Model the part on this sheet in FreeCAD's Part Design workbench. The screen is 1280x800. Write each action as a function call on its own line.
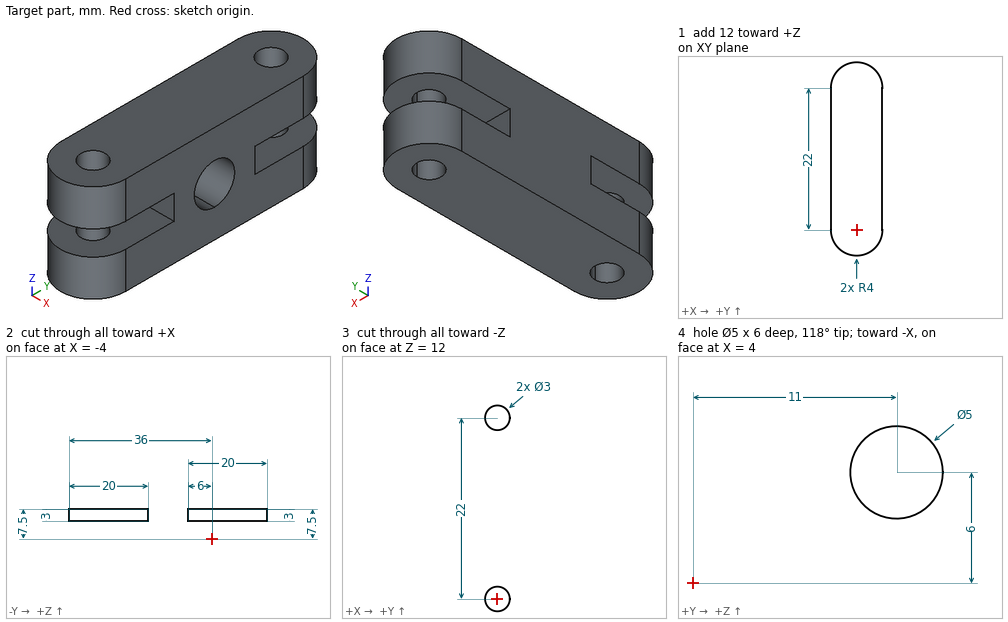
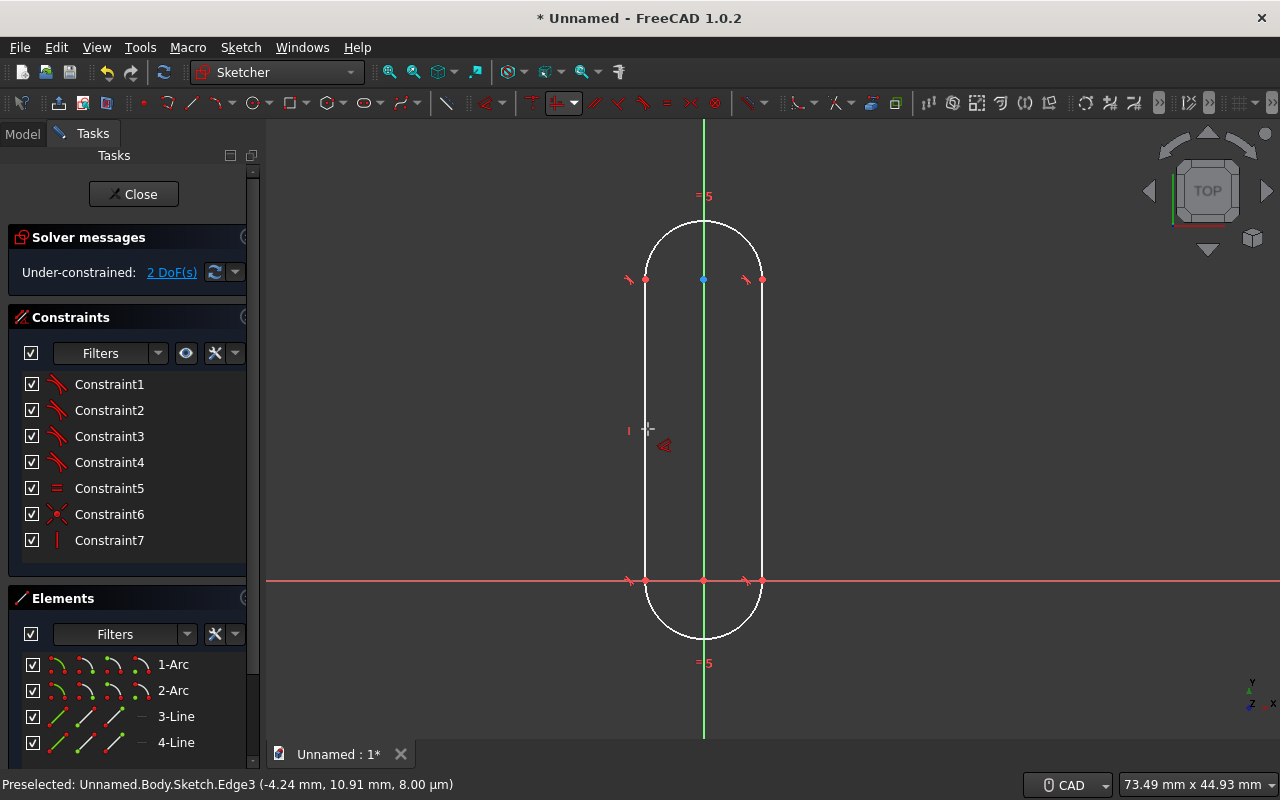
click(669, 628)
click(650, 654)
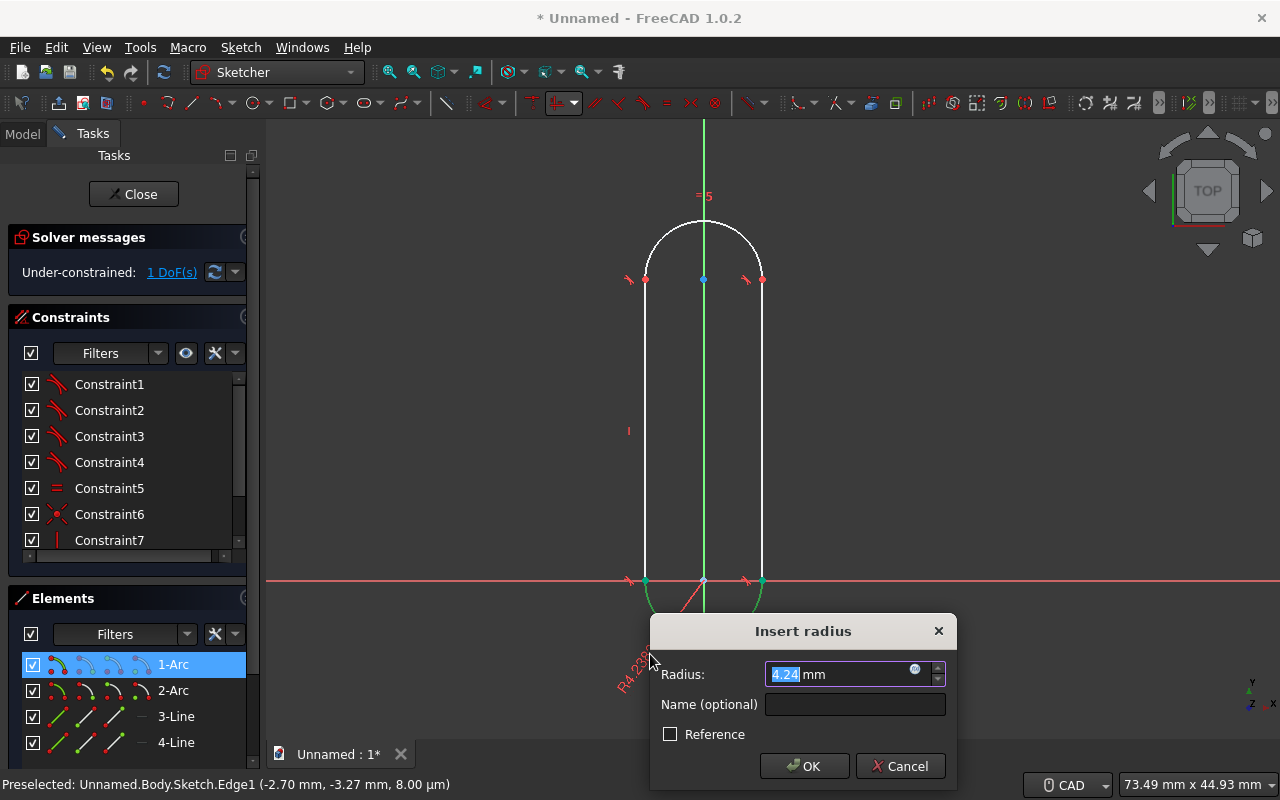
text(4)
key(Return)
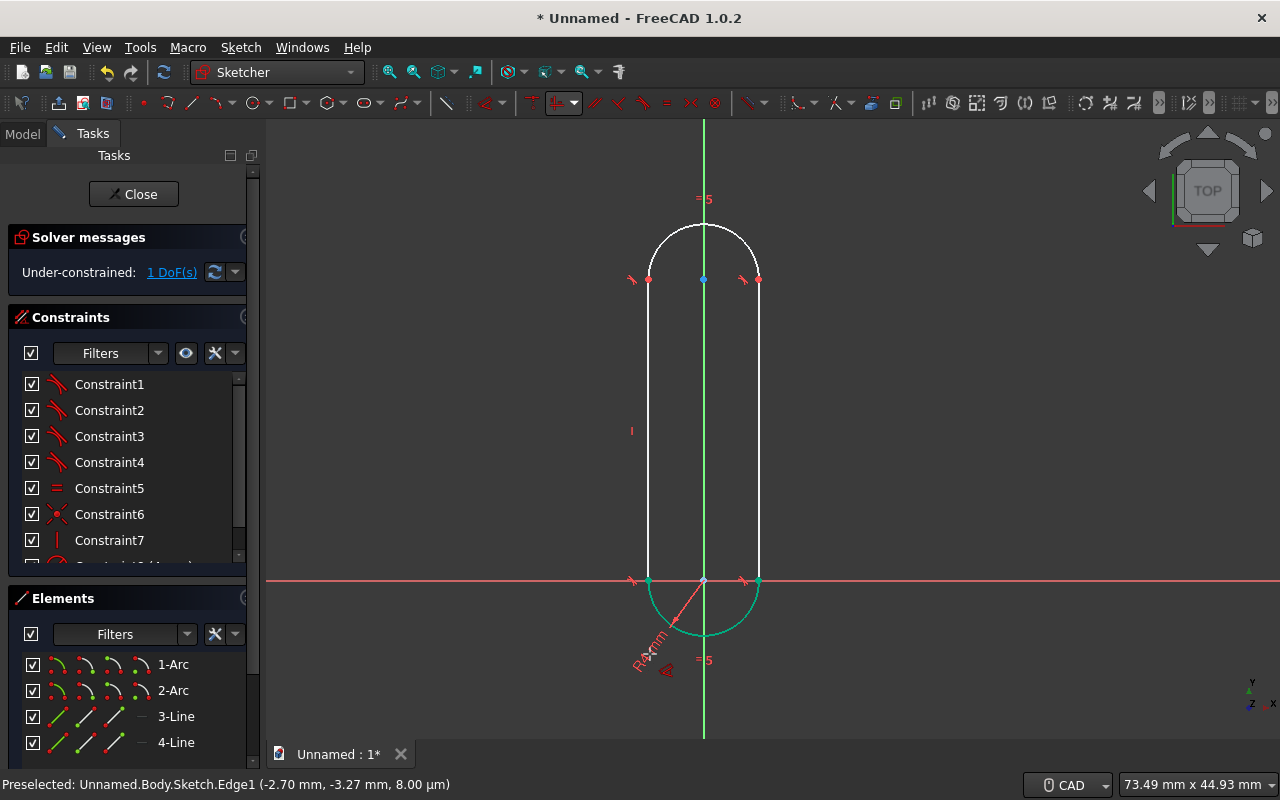
click(648, 490)
click(614, 430)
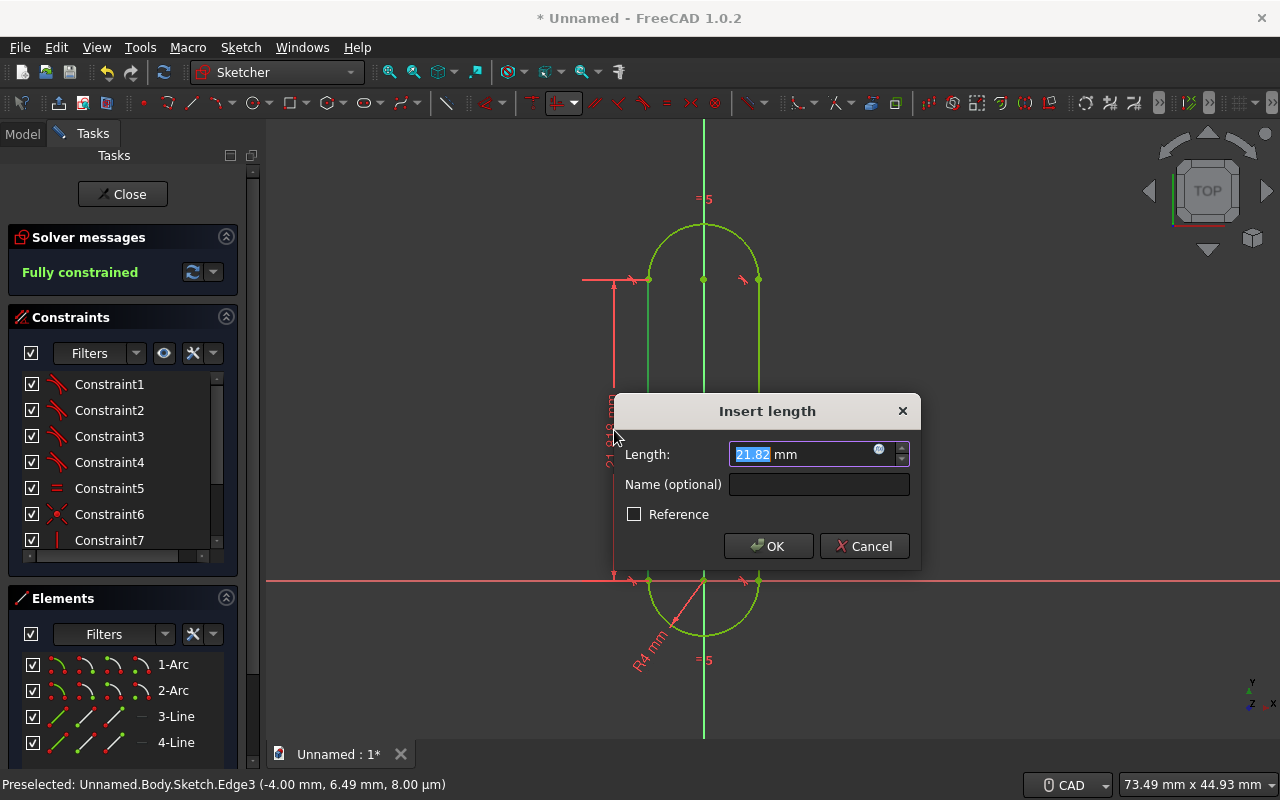
text(22)
key(Return)
key(Escape)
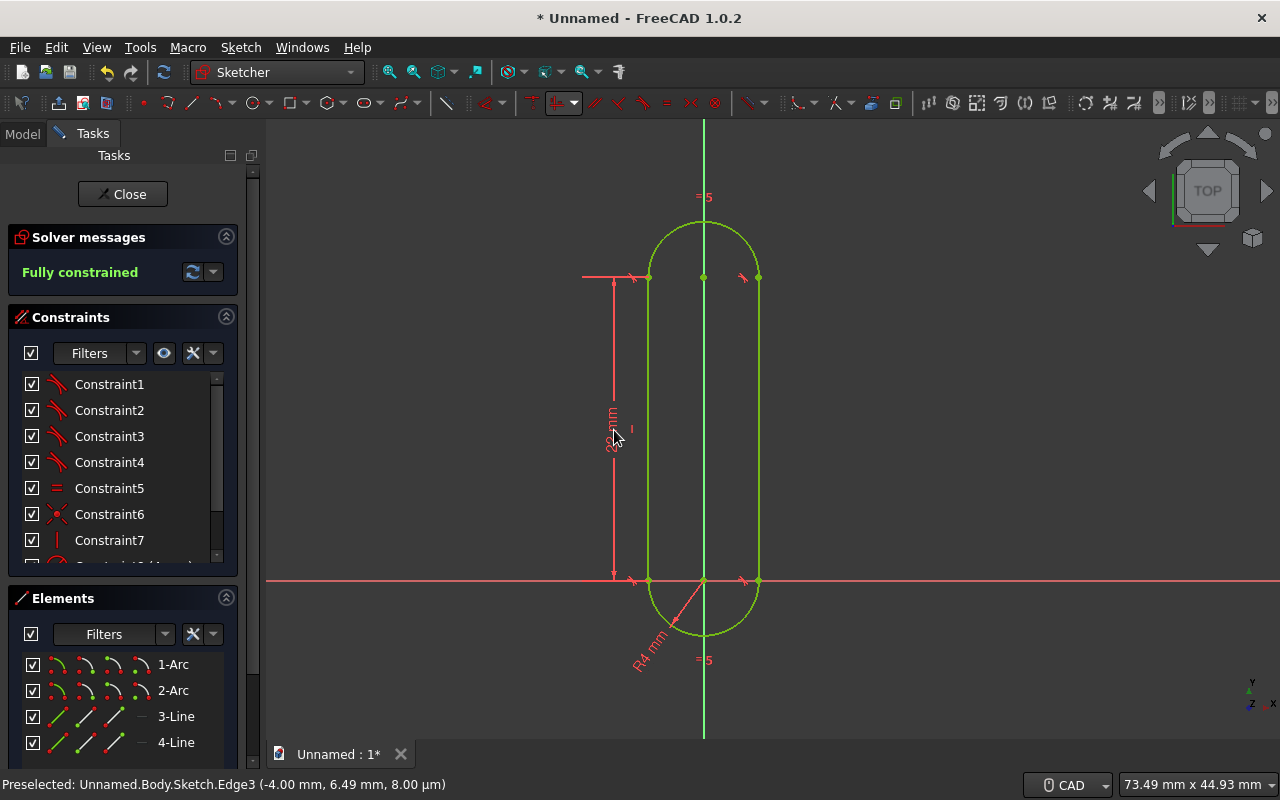
click(123, 194)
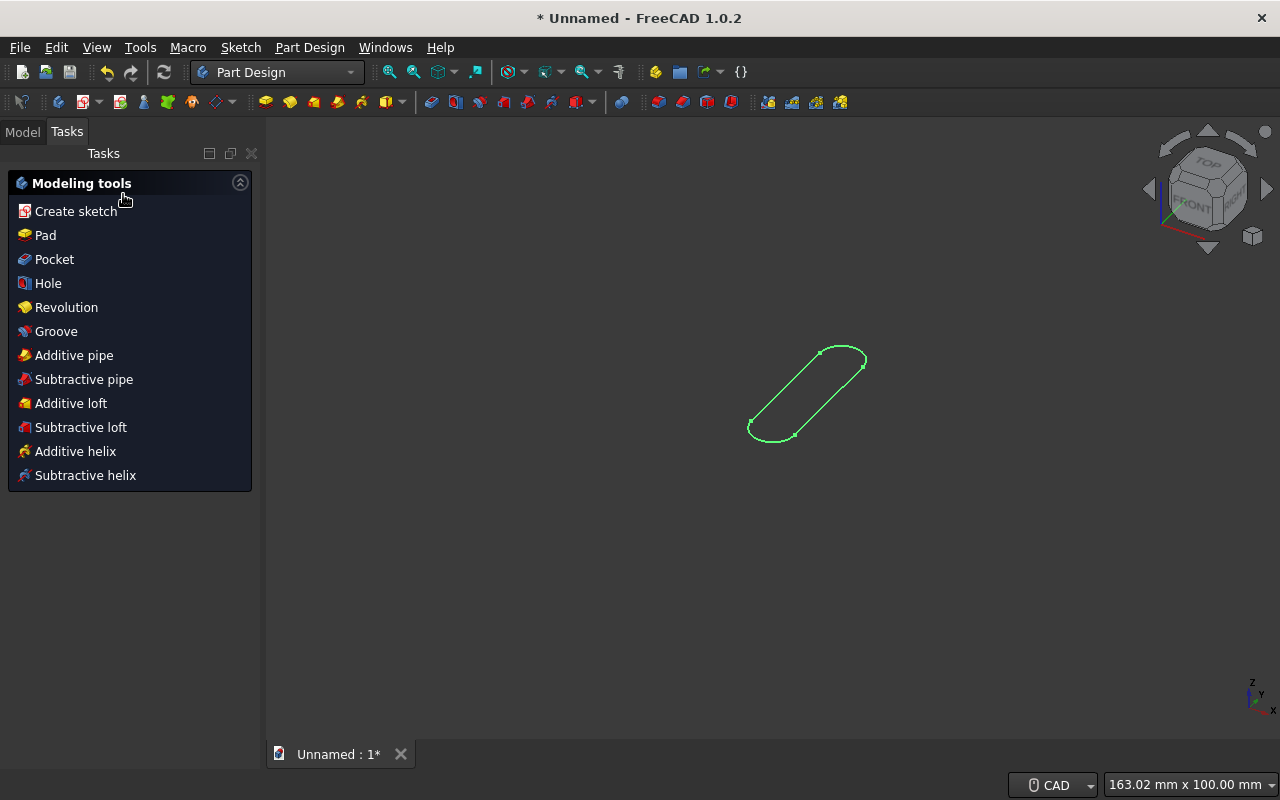
click(266, 102)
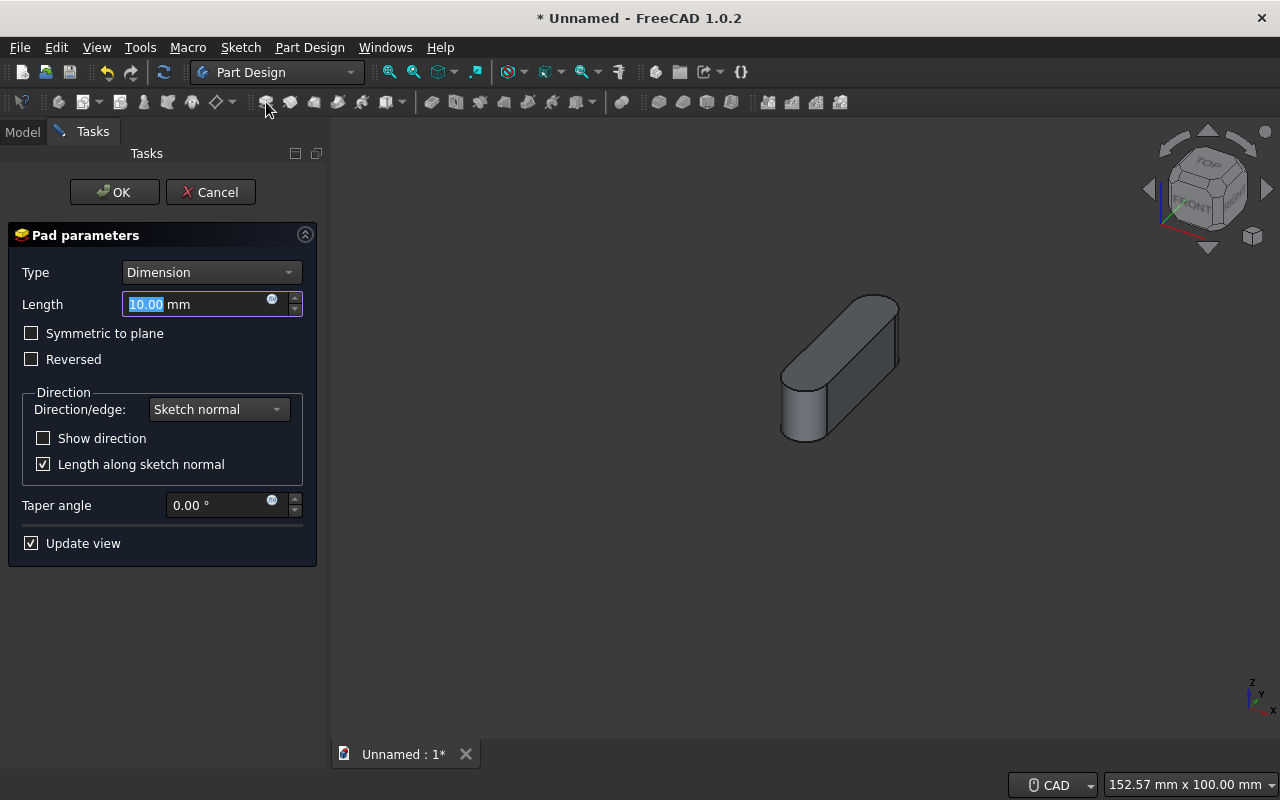
text(12)
key(Tab)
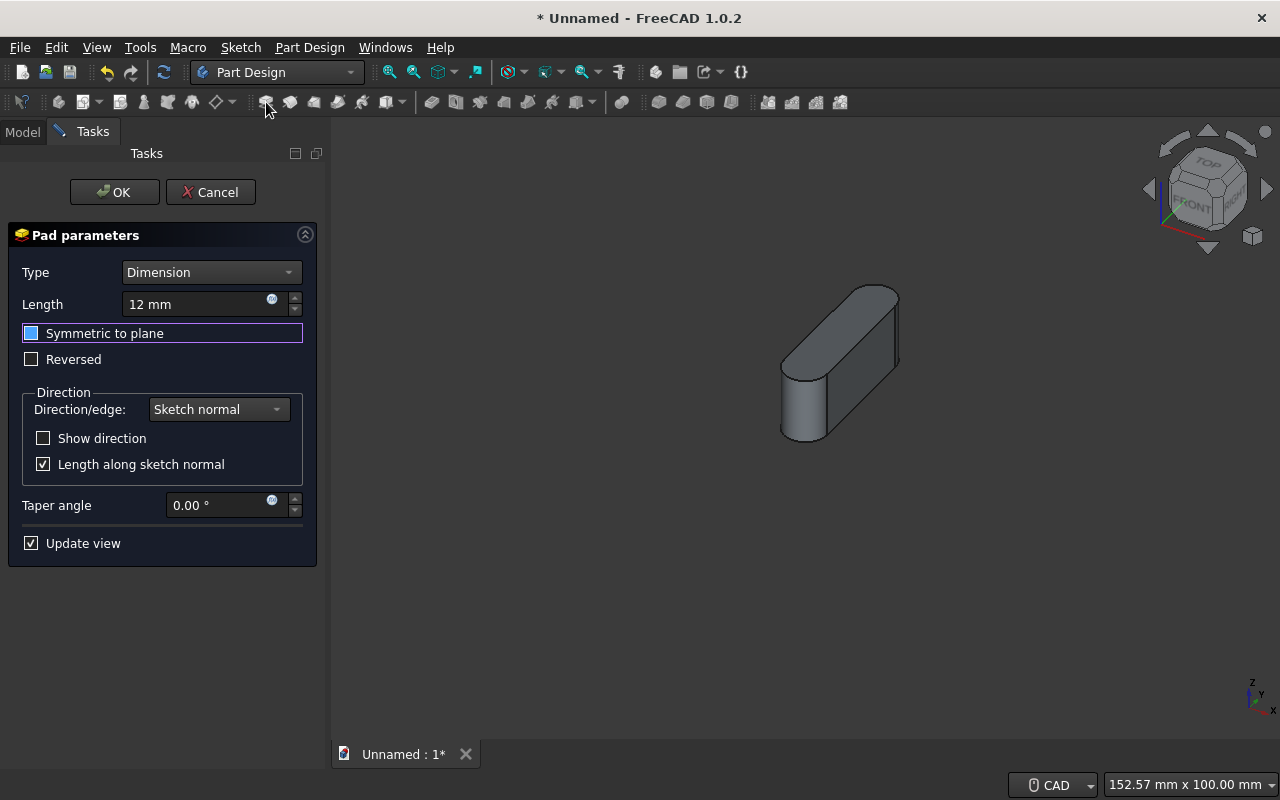
click(115, 192)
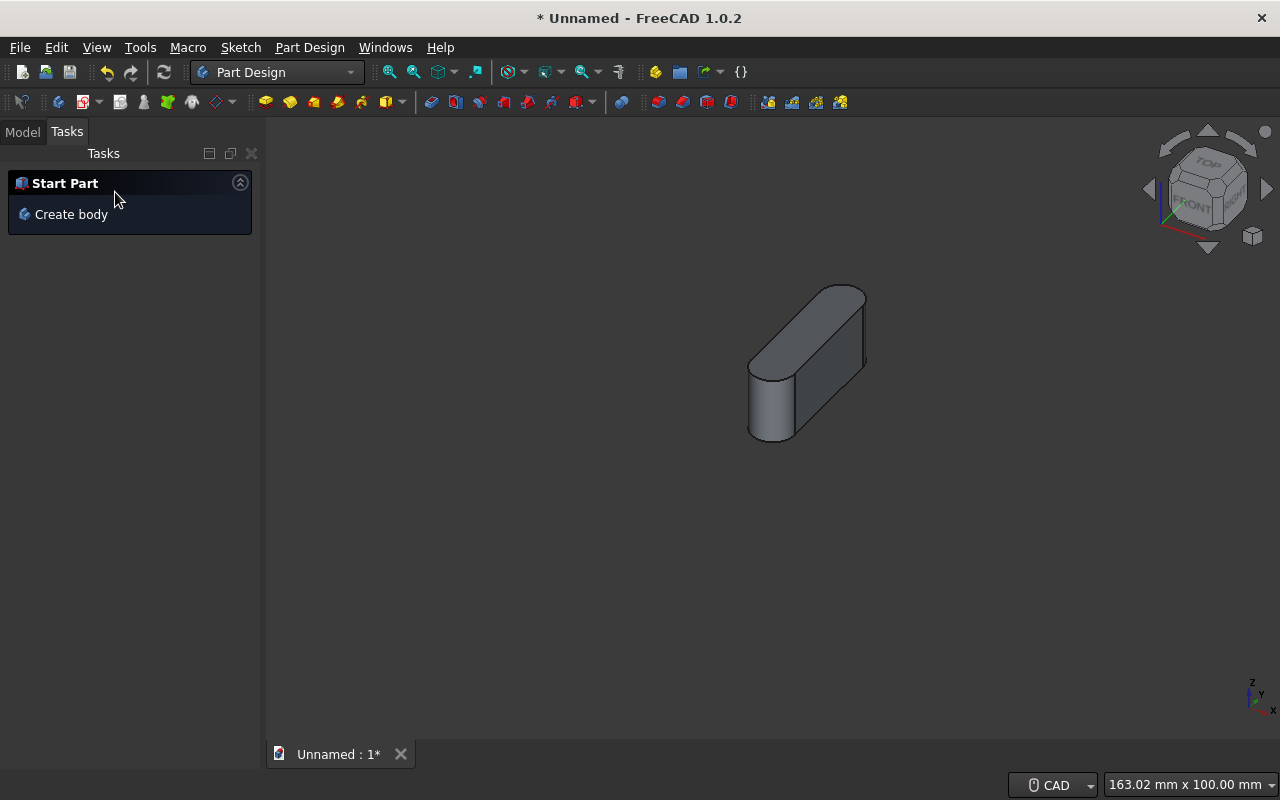
key(v)
key(f)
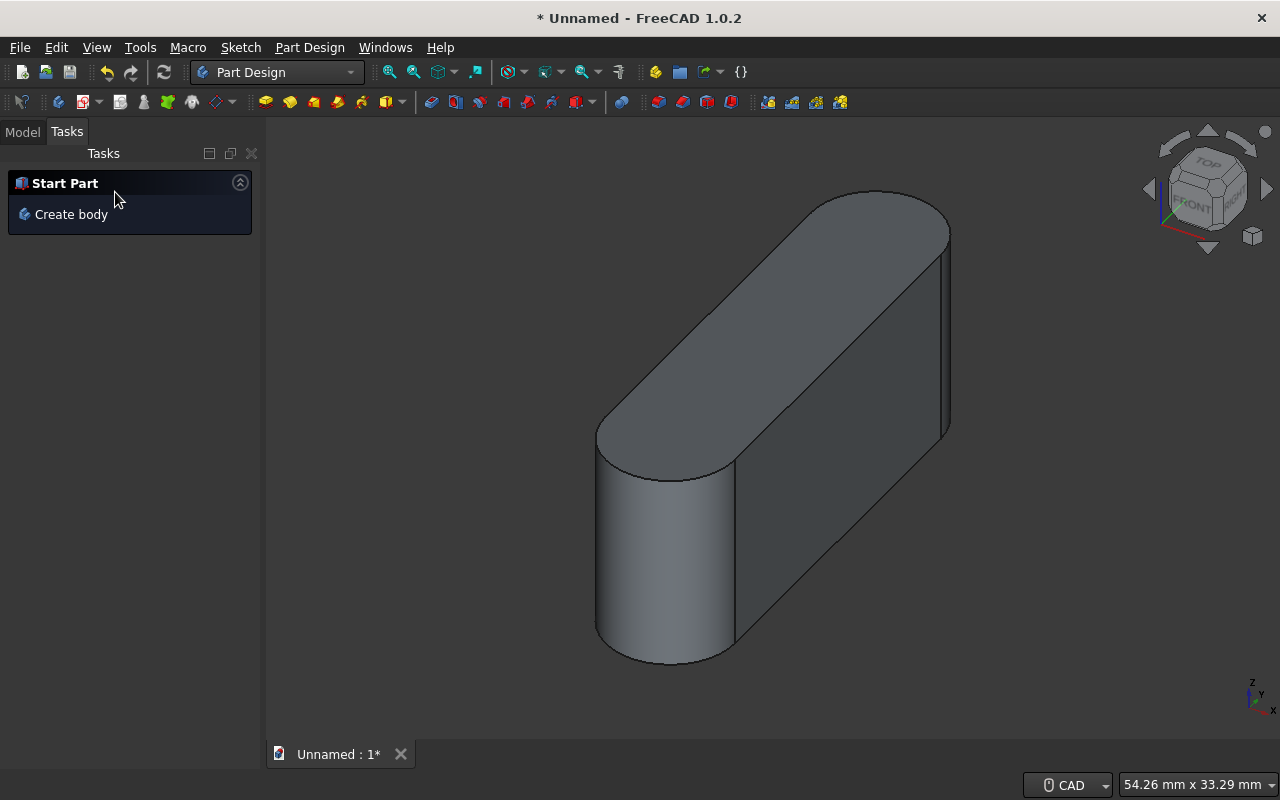
key(6)